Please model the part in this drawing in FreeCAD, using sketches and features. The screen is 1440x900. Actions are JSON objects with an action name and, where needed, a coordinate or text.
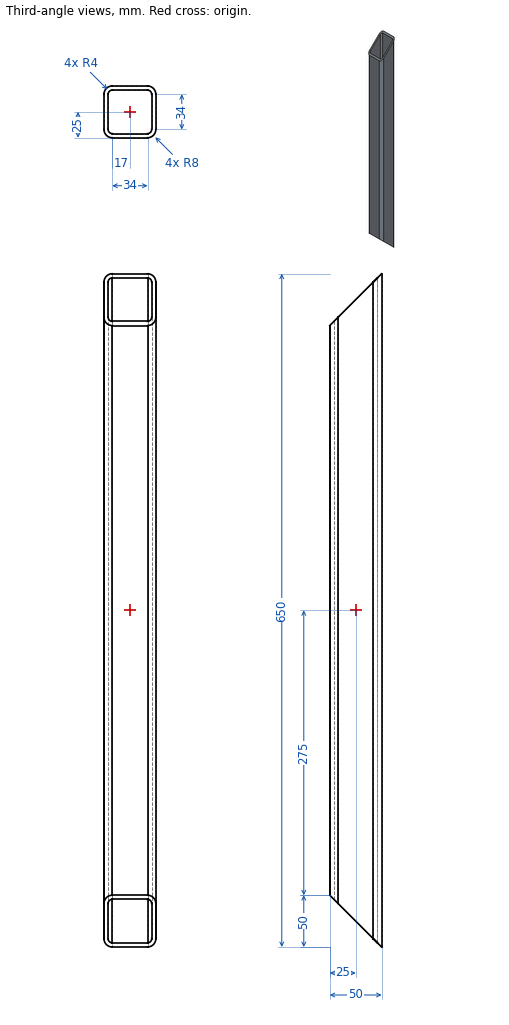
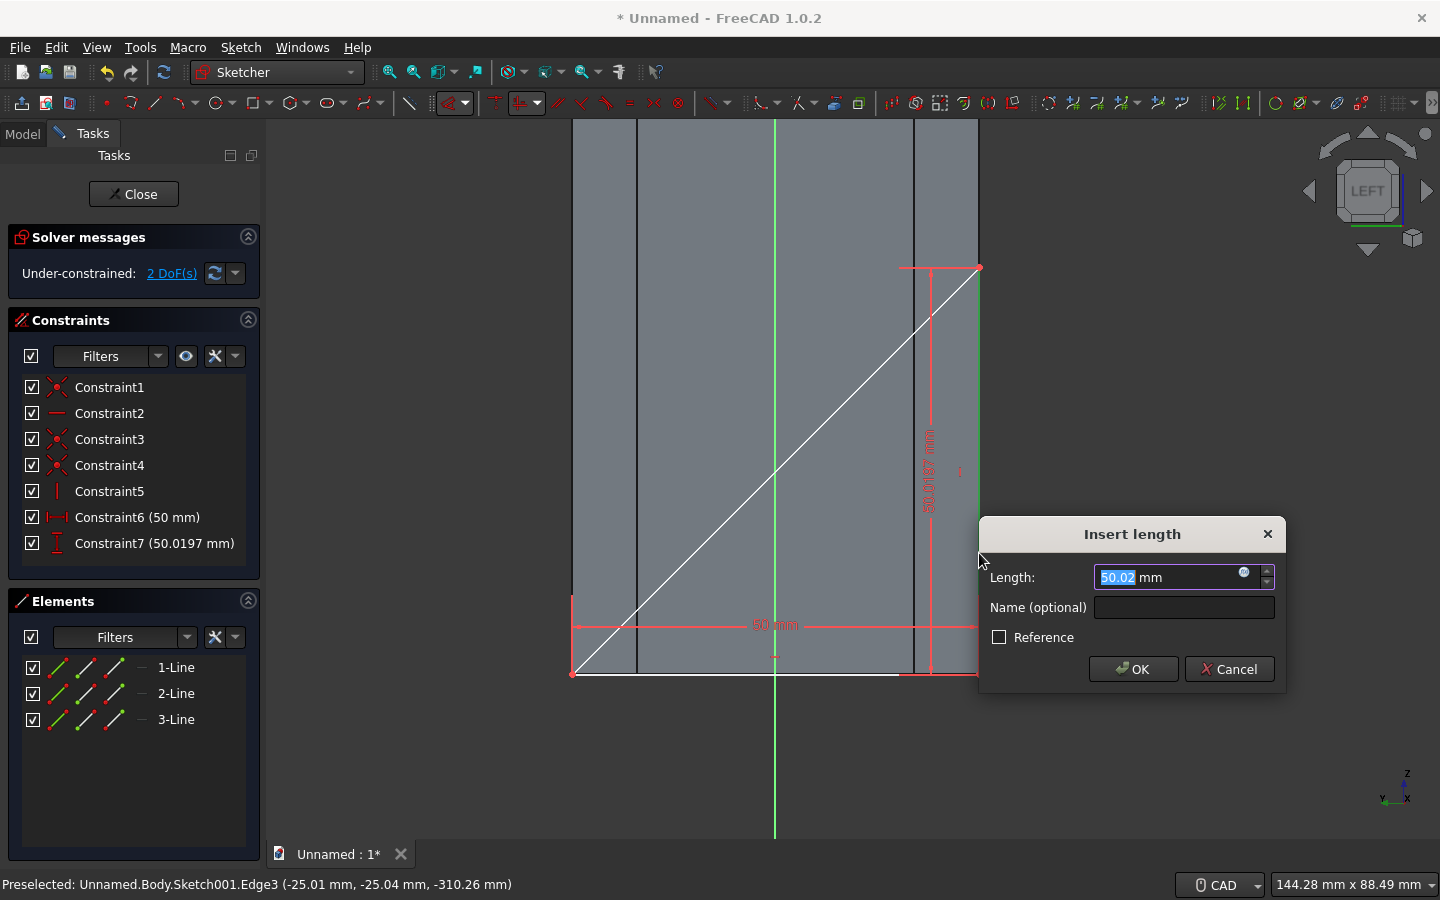
{"action": "type", "text": "50"}
{"action": "key", "text": "Return"}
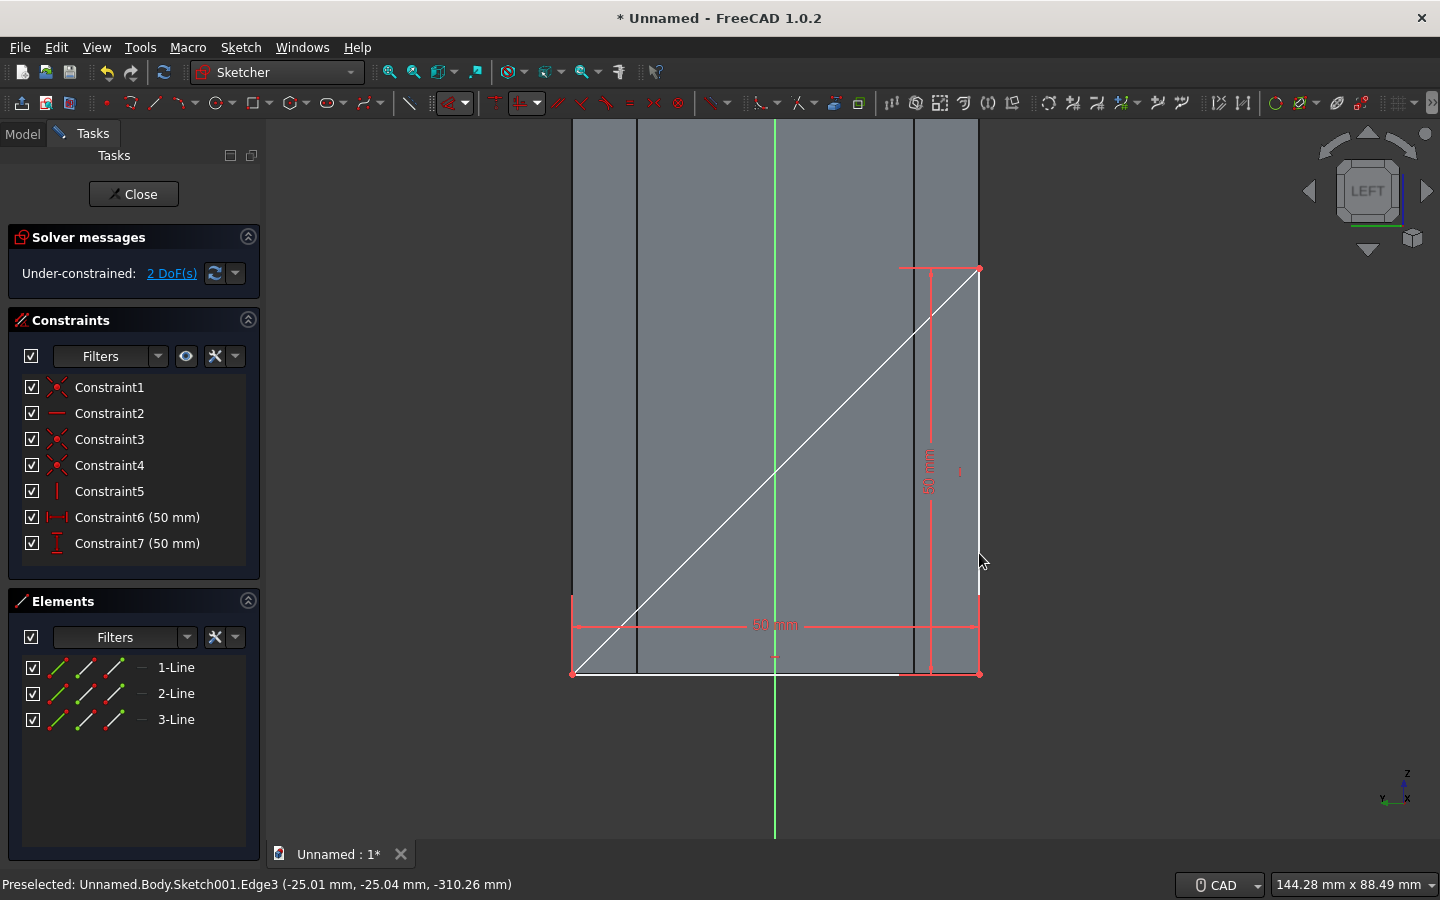
{"action": "left_click", "coordinate": [979, 268]}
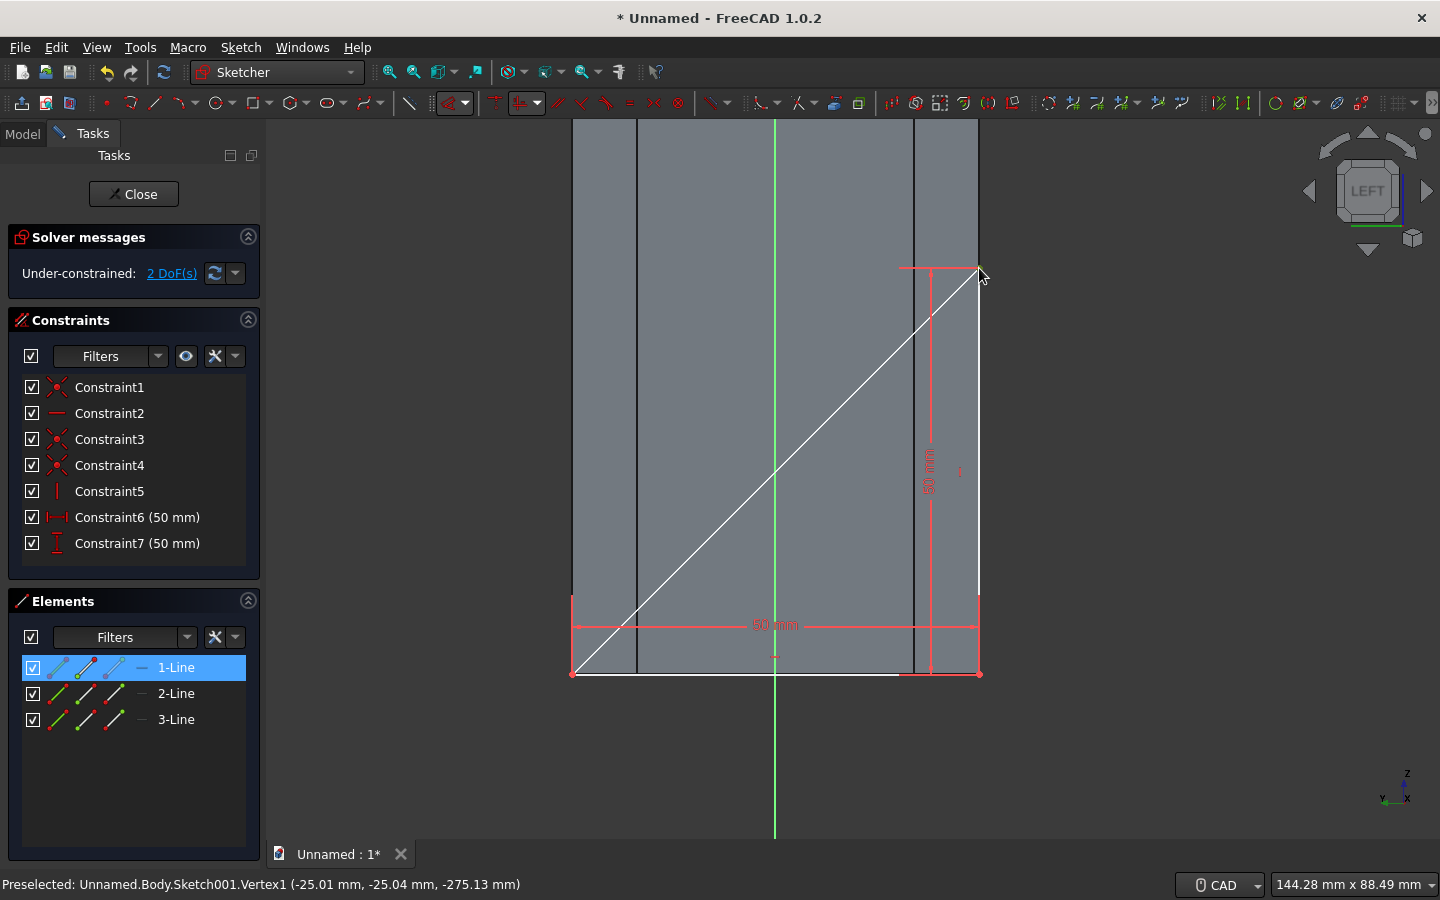
{"action": "left_click", "coordinate": [468, 104]}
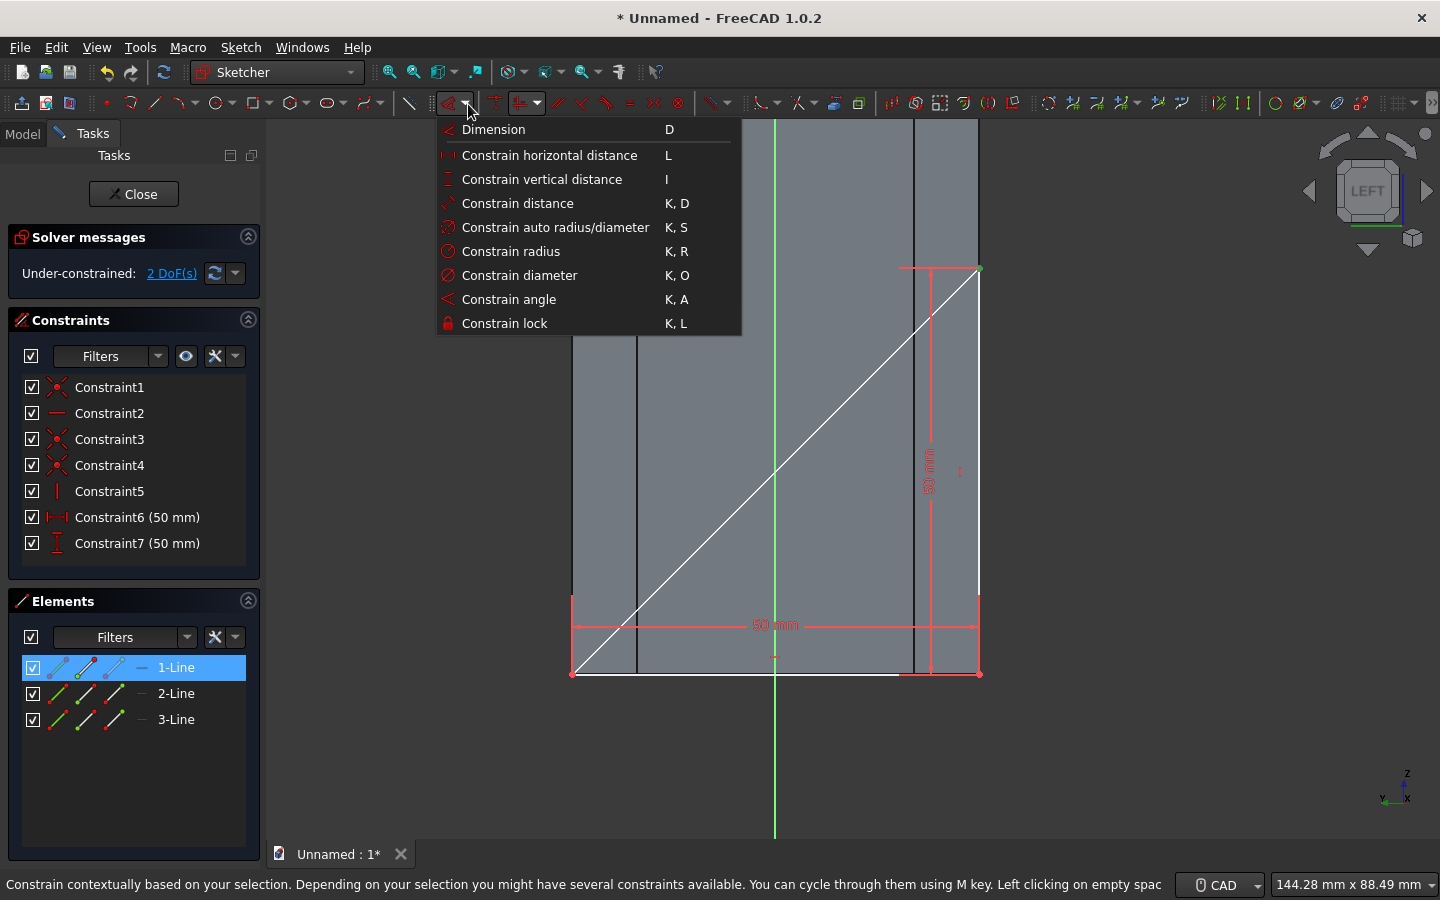
{"action": "left_click", "coordinate": [589, 155]}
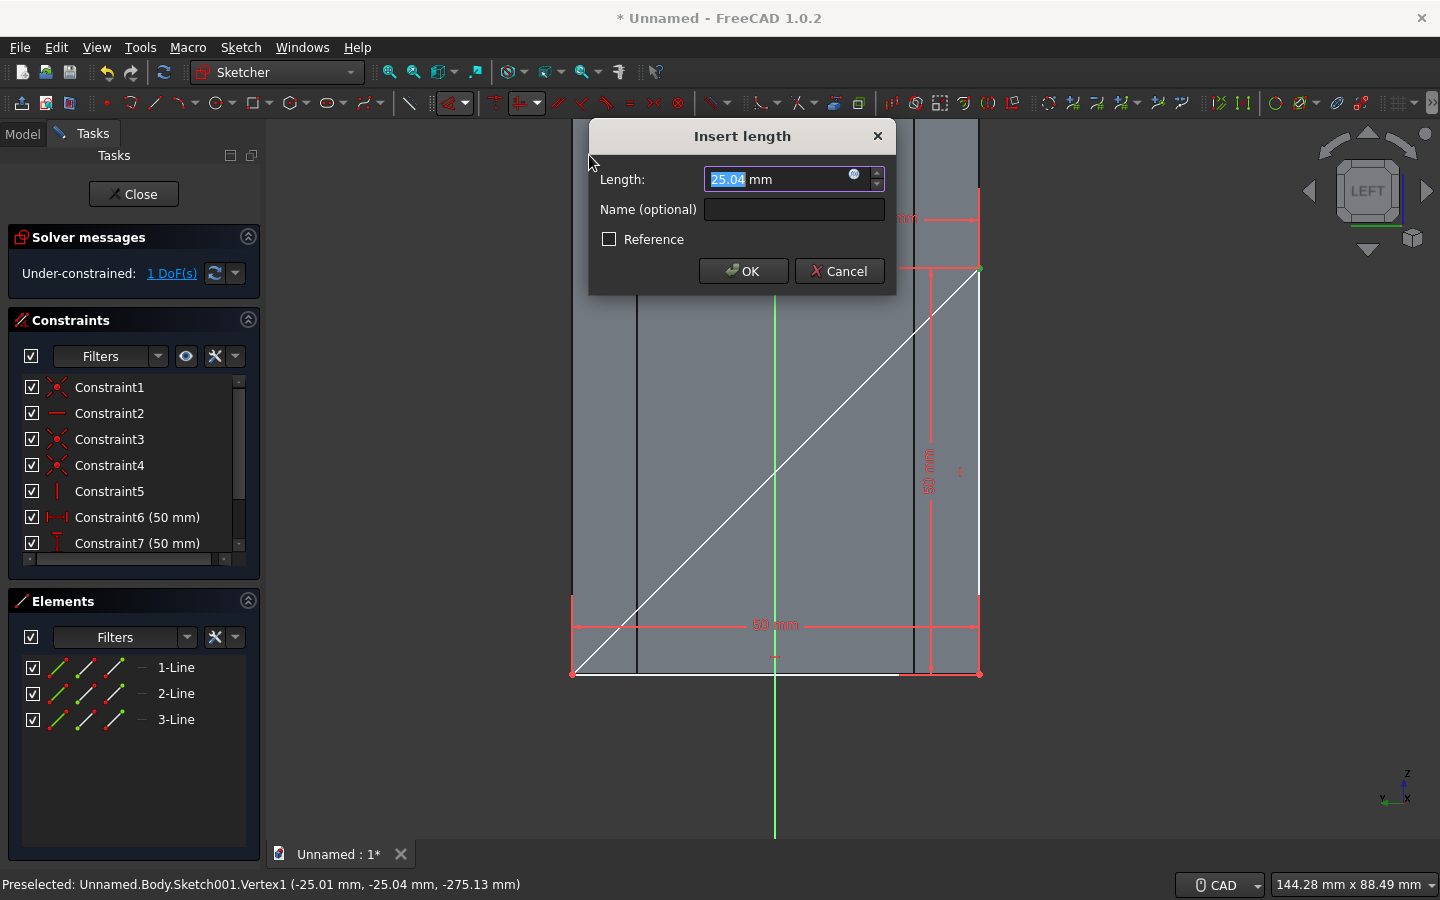
{"action": "type", "text": "25"}
{"action": "key", "text": "Return"}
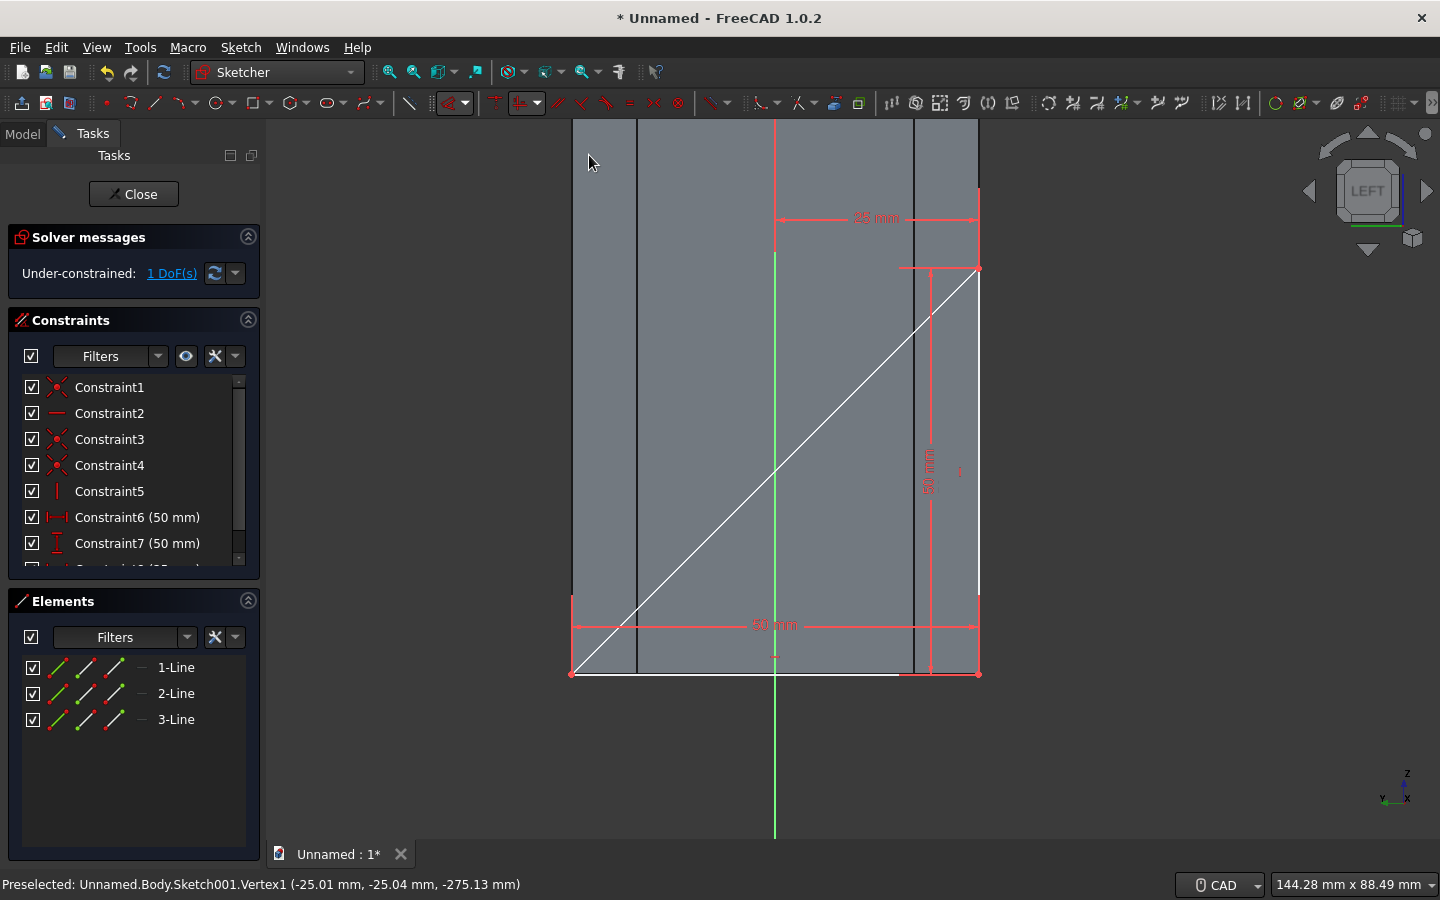
{"action": "left_click", "coordinate": [979, 268]}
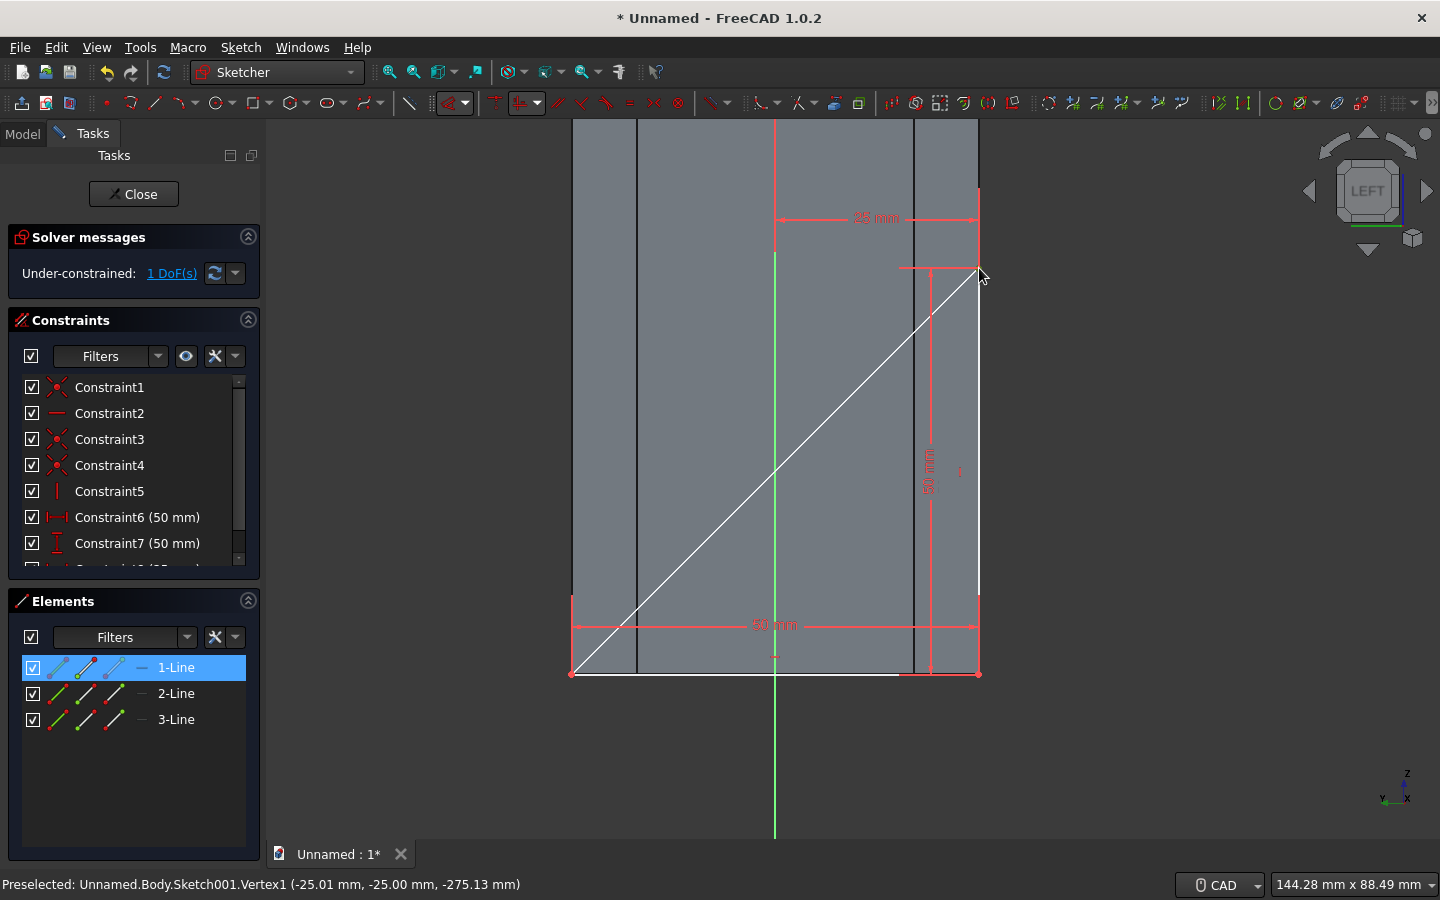
{"action": "key", "text": "i"}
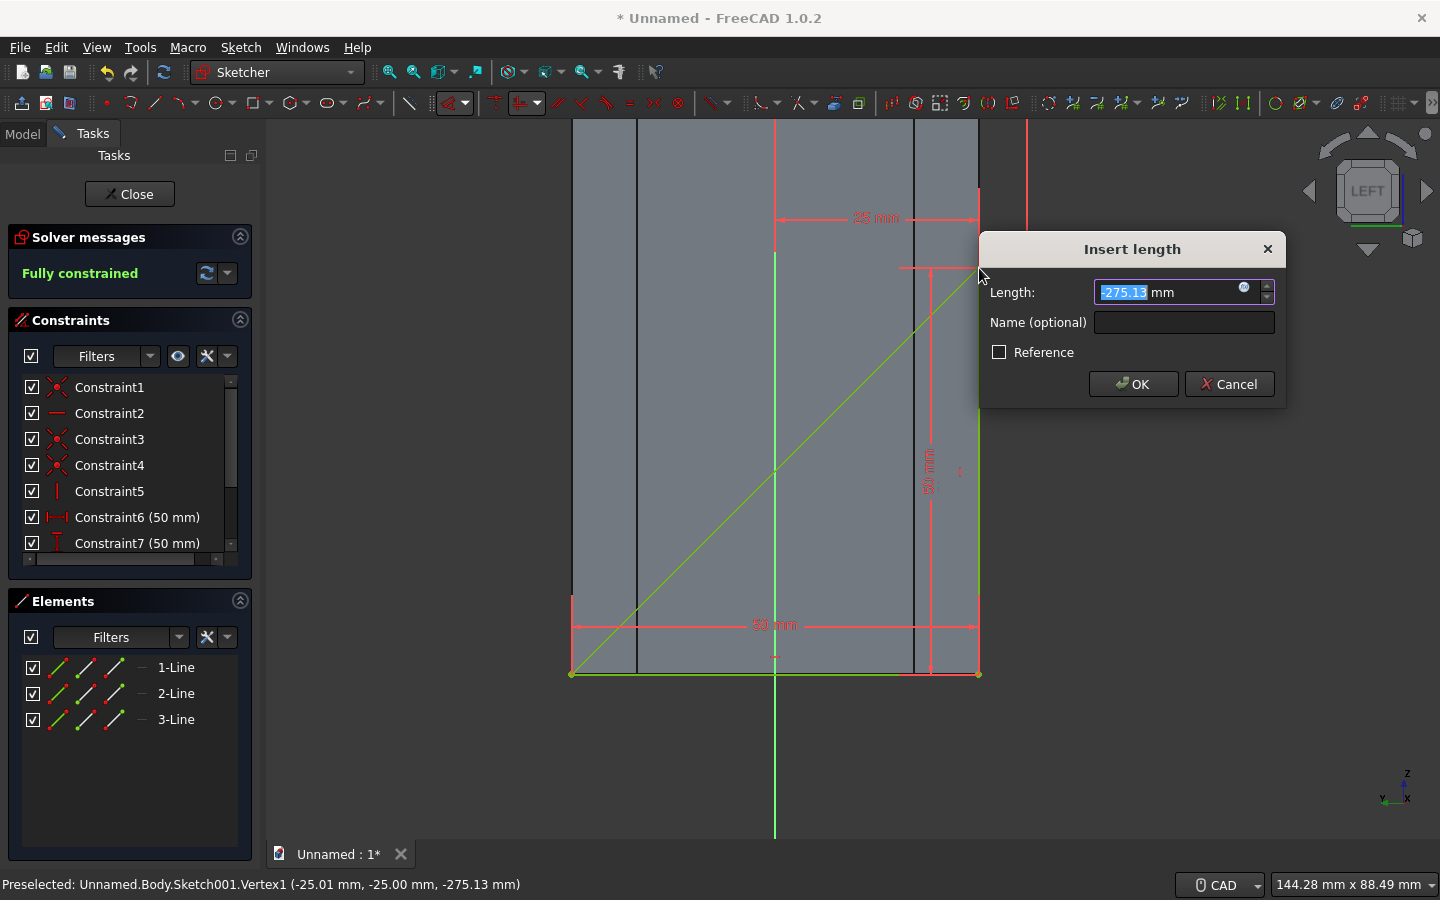
{"action": "type", "text": "-275"}
{"action": "key", "text": "Return"}